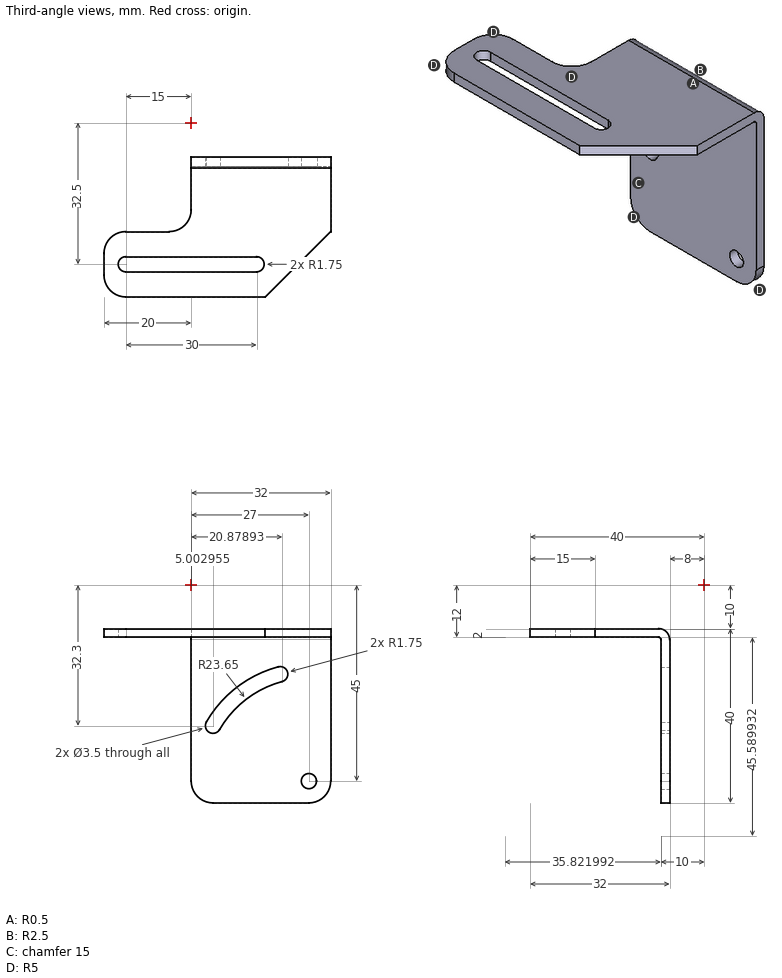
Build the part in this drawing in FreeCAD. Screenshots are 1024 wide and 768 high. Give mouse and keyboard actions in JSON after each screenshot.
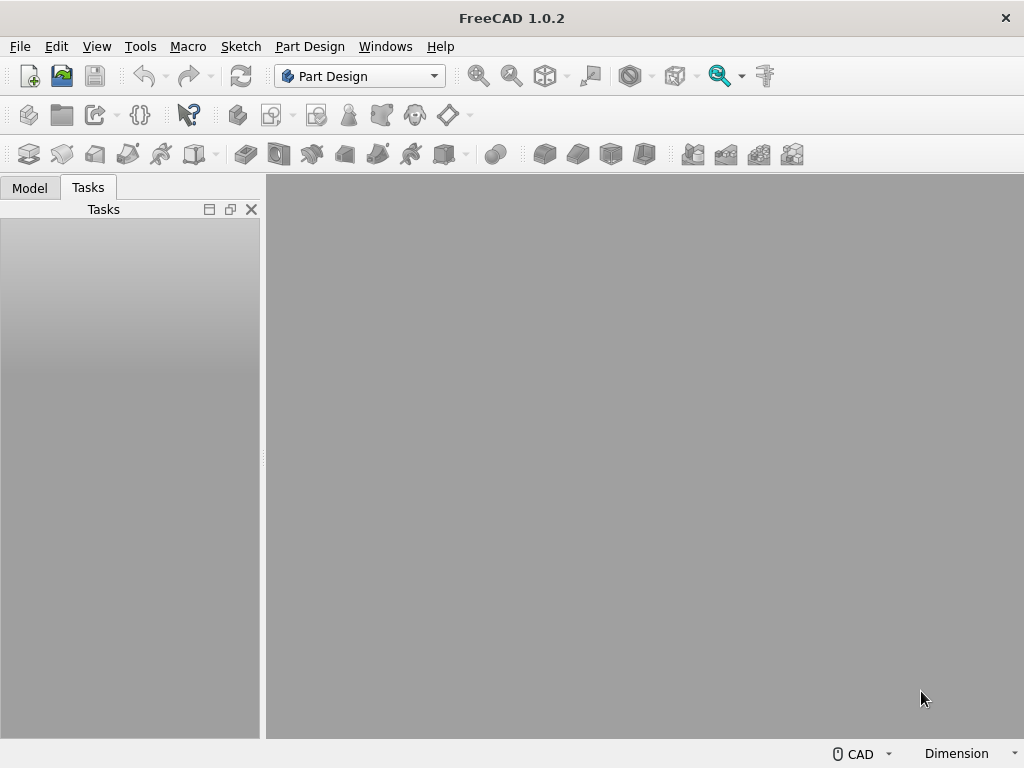
{"action": "left_click", "coordinate": [29, 76]}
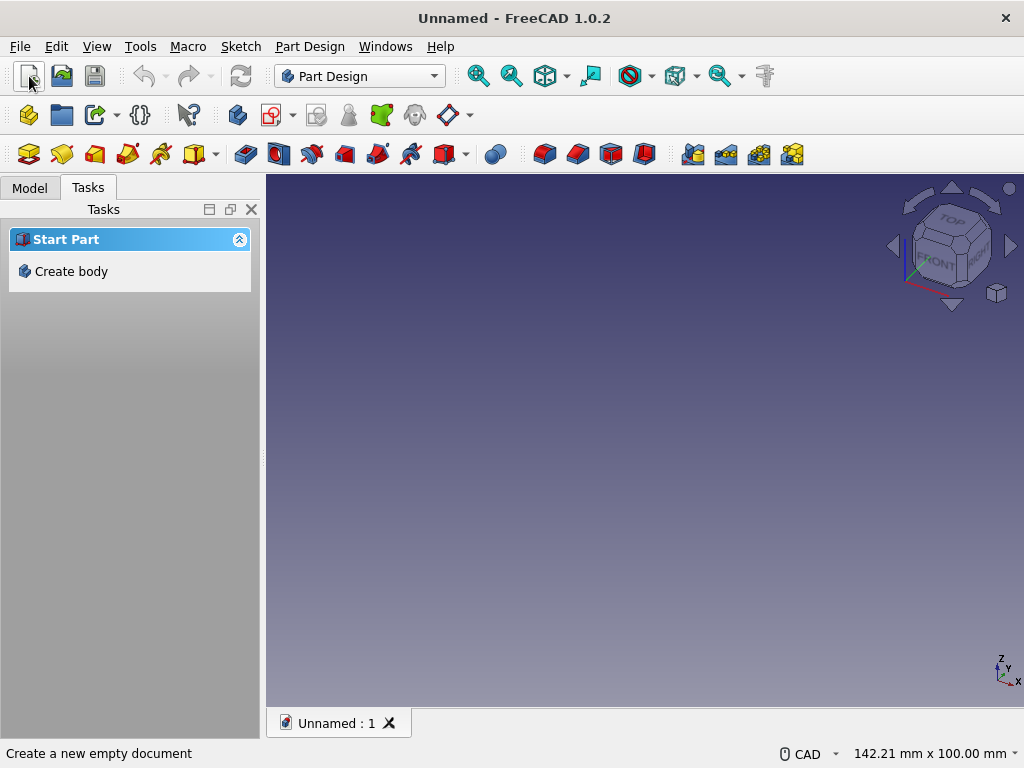
{"action": "left_click", "coordinate": [270, 116]}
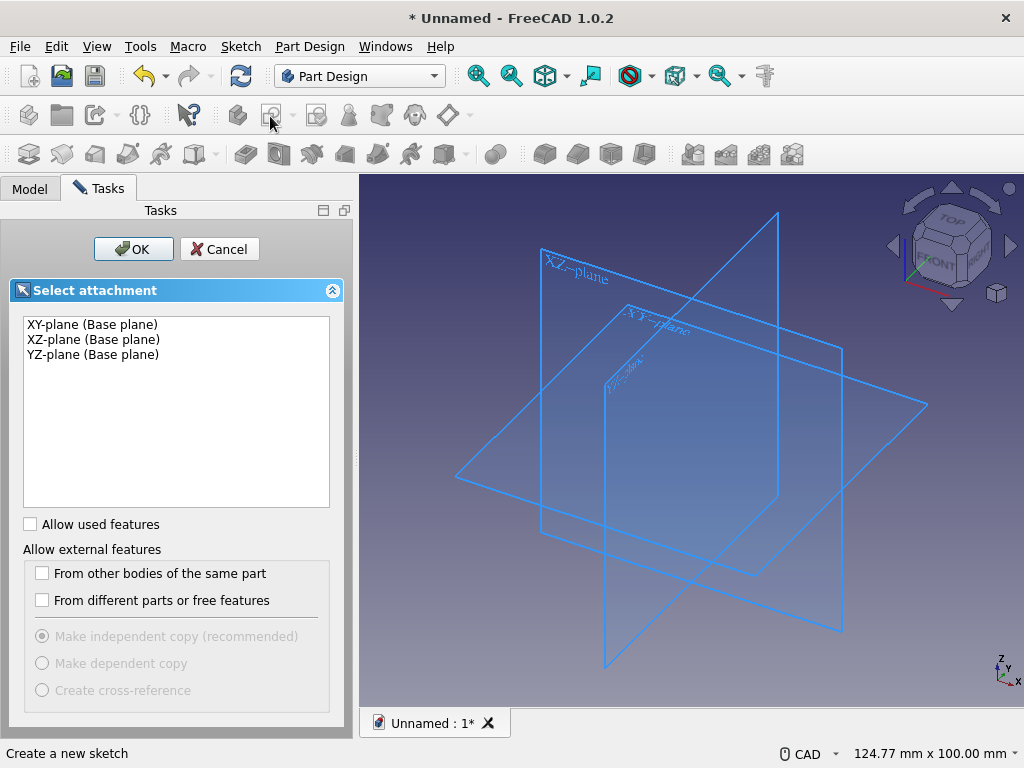
{"action": "left_click", "coordinate": [84, 354]}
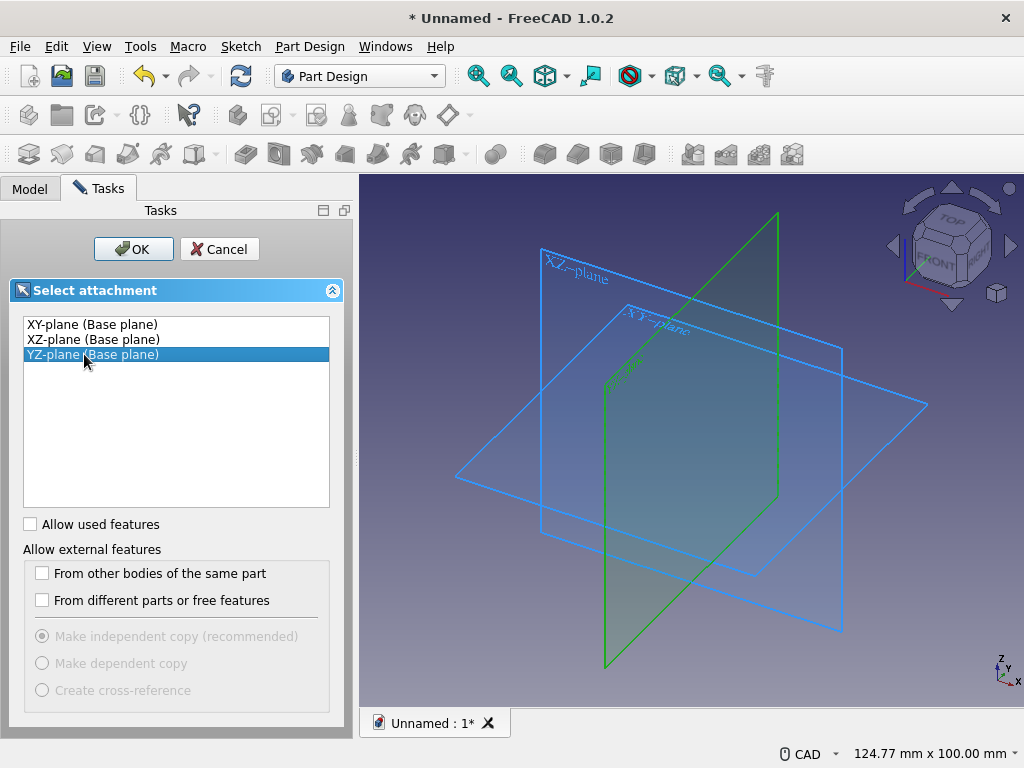
{"action": "left_click", "coordinate": [134, 249]}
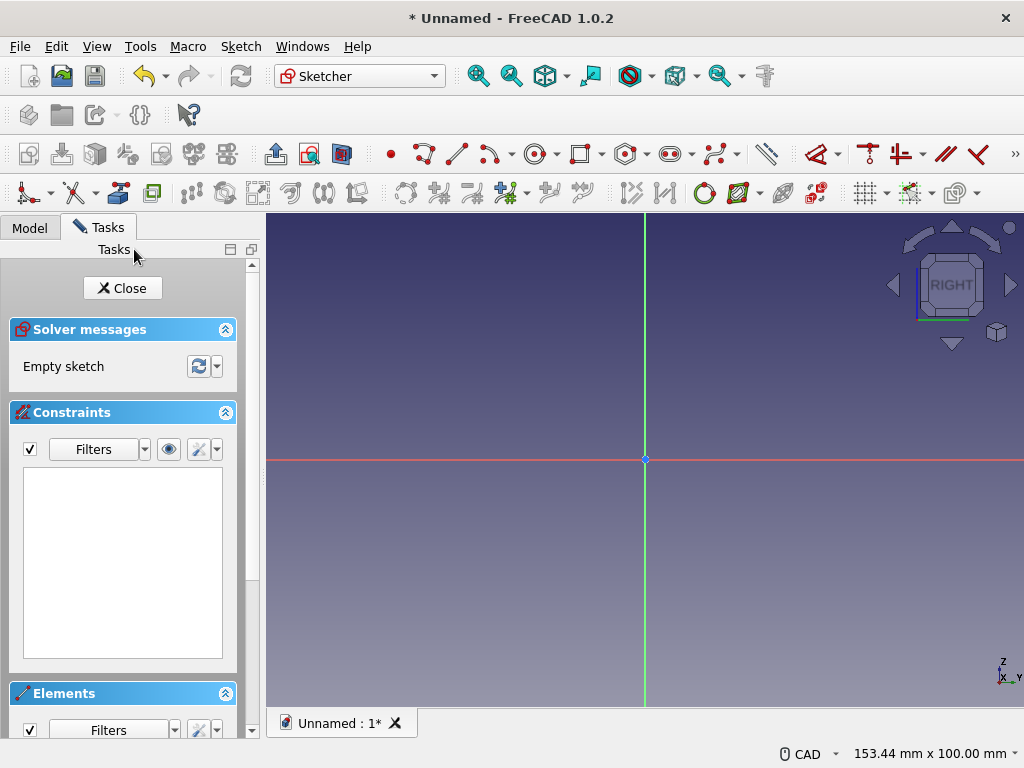
{"action": "scroll", "coordinate": [713, 241], "scroll_direction": "down", "scroll_amount": 1}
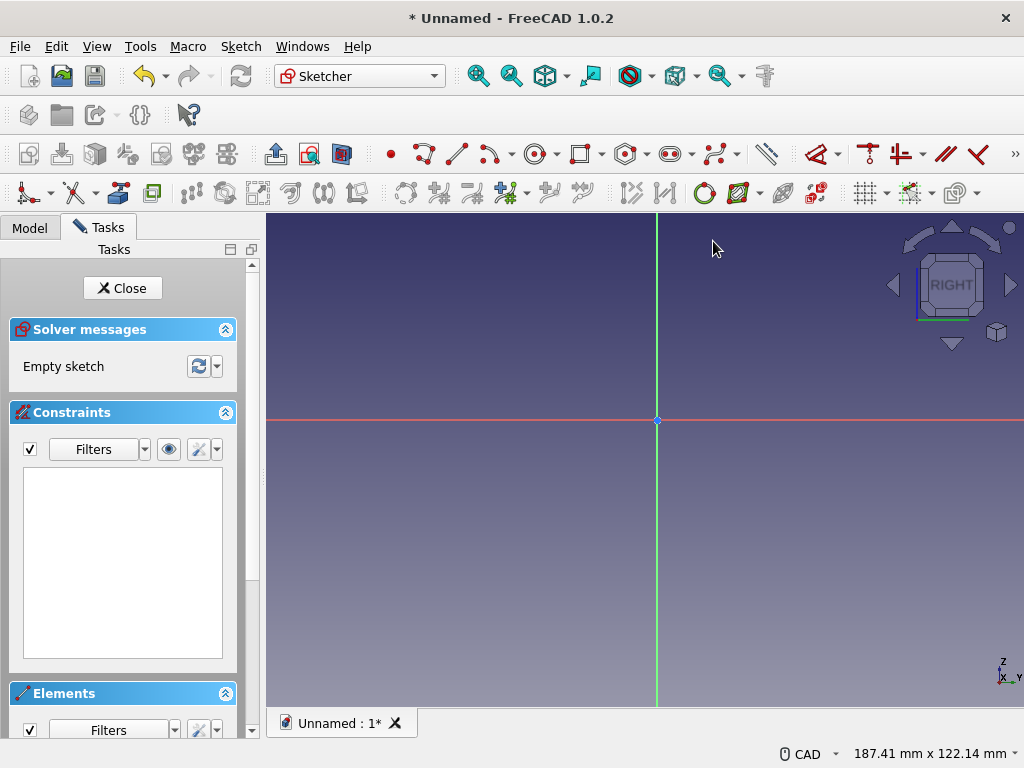
{"action": "scroll", "coordinate": [577, 646], "scroll_direction": "up", "scroll_amount": 2}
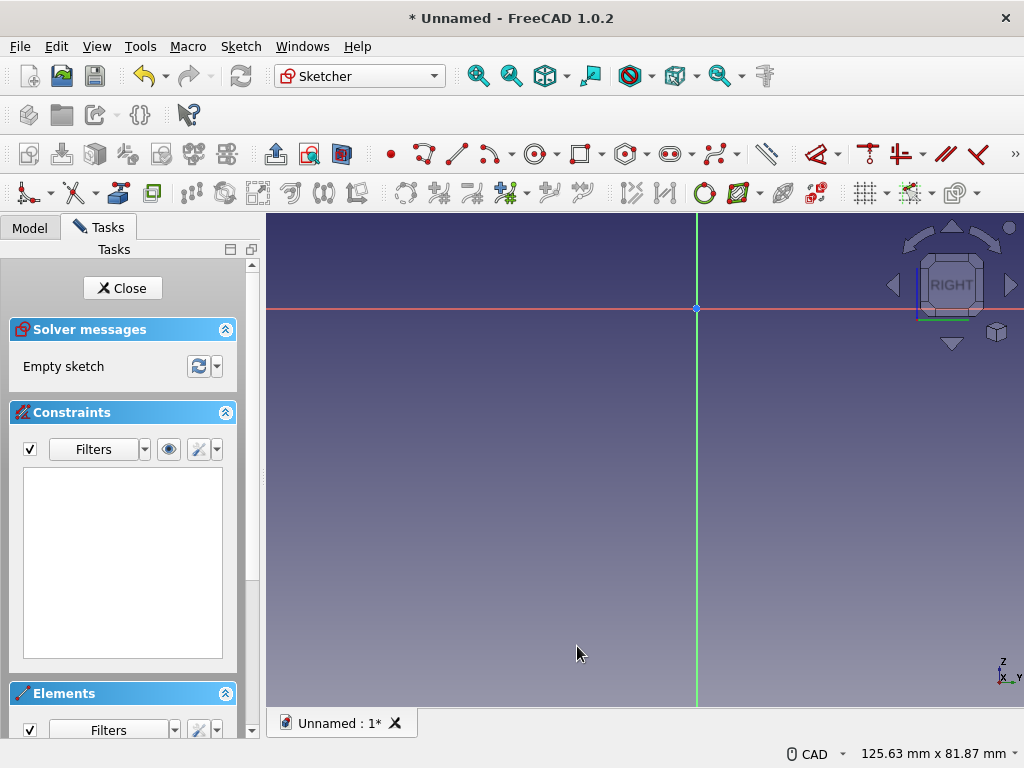
{"action": "key", "text": "g r"}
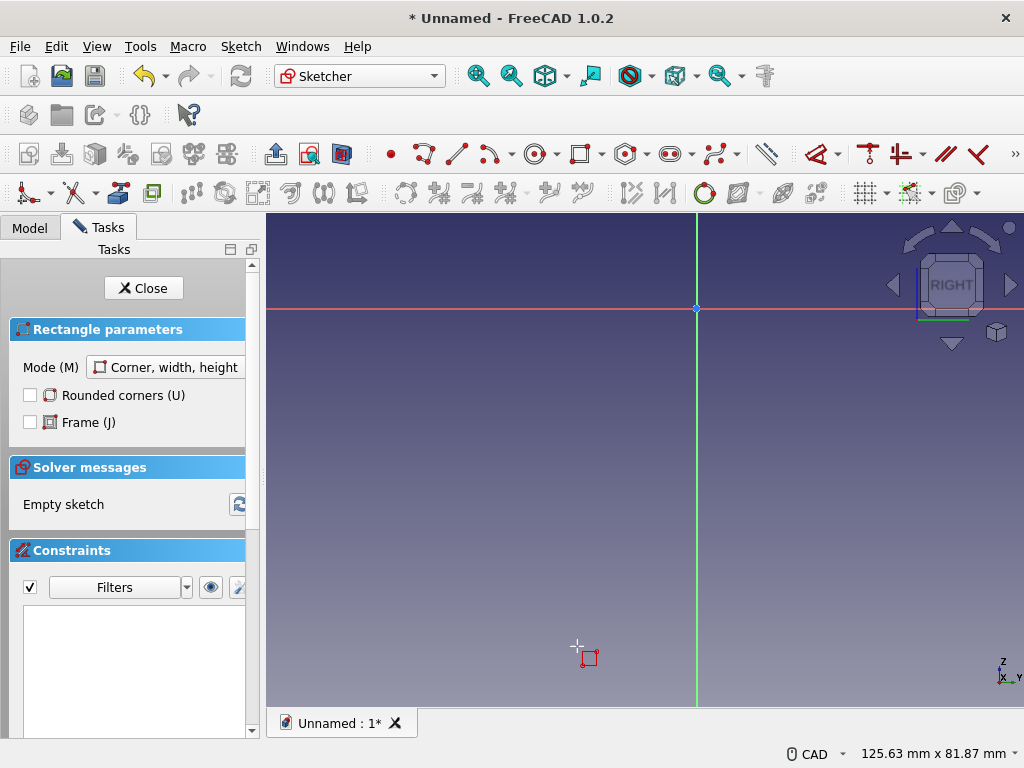
{"action": "left_click", "coordinate": [455, 369]}
{"action": "mouse_move", "coordinate": [649, 611]}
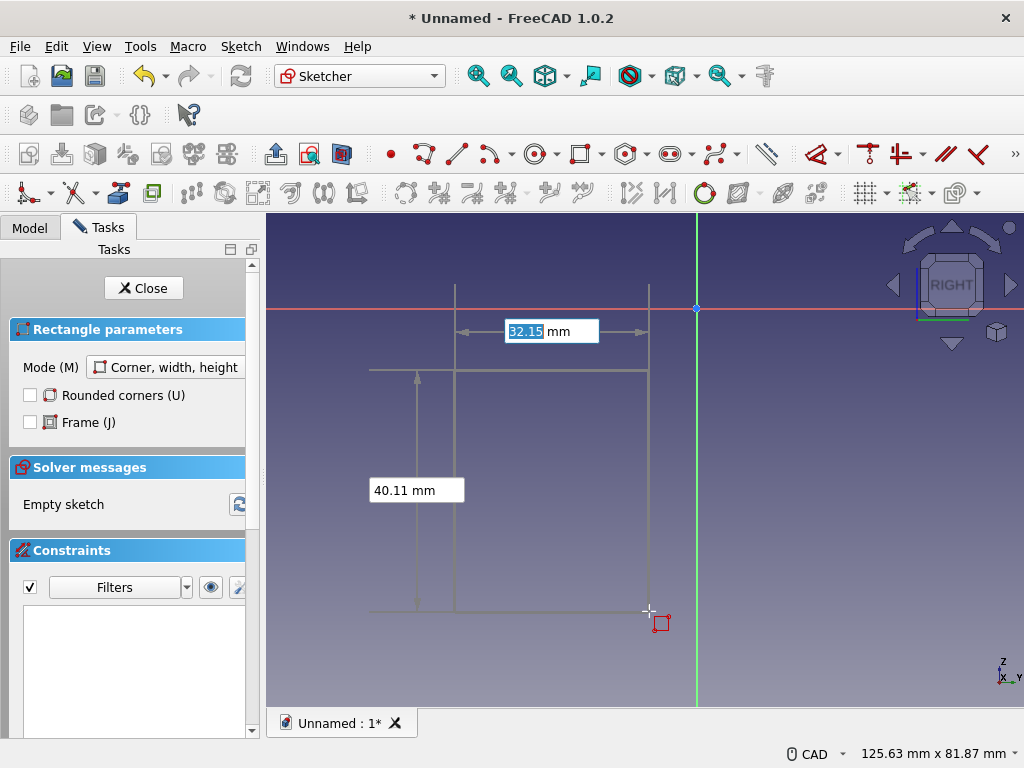
{"action": "type", "text": "32"}
{"action": "key", "text": "Tab"}
{"action": "type", "text": "40"}
{"action": "key", "text": "Return"}
{"action": "key", "text": "Escape"}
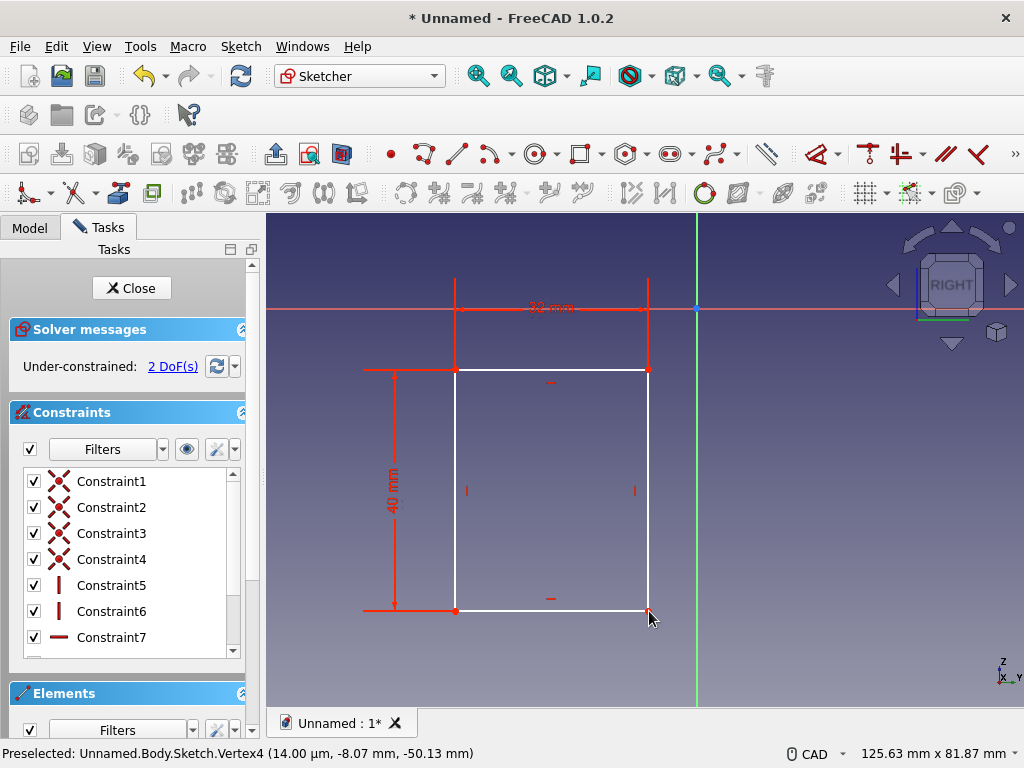
{"action": "key", "text": "d"}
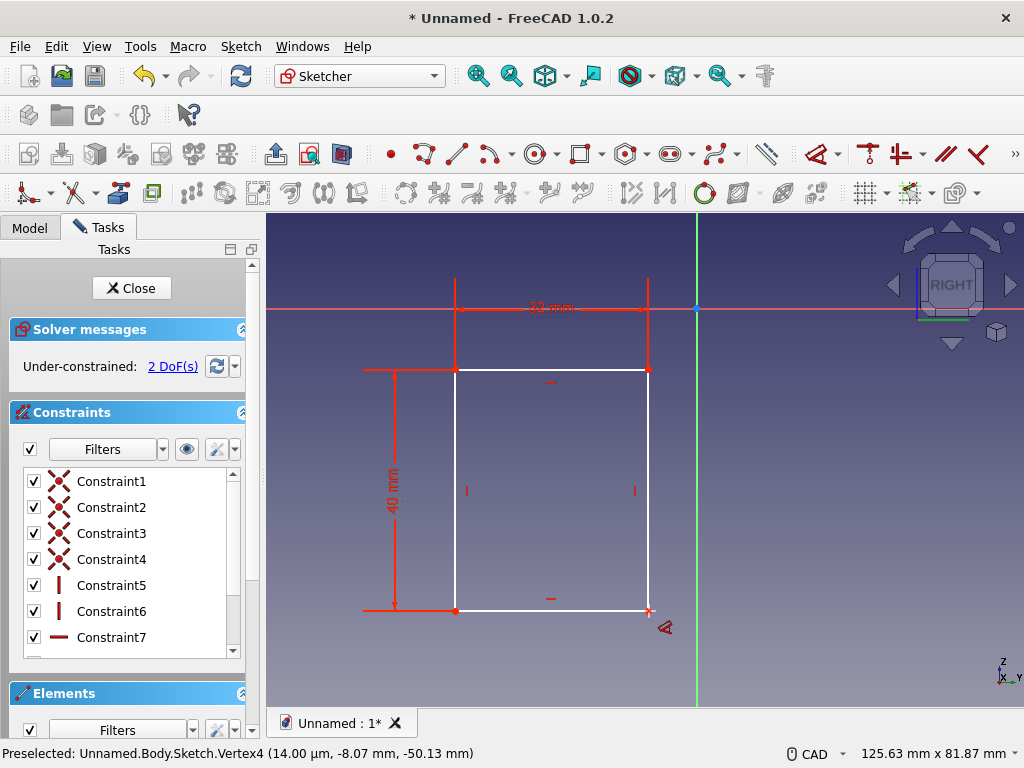
{"action": "left_click", "coordinate": [648, 611]}
{"action": "left_click", "coordinate": [672, 645]}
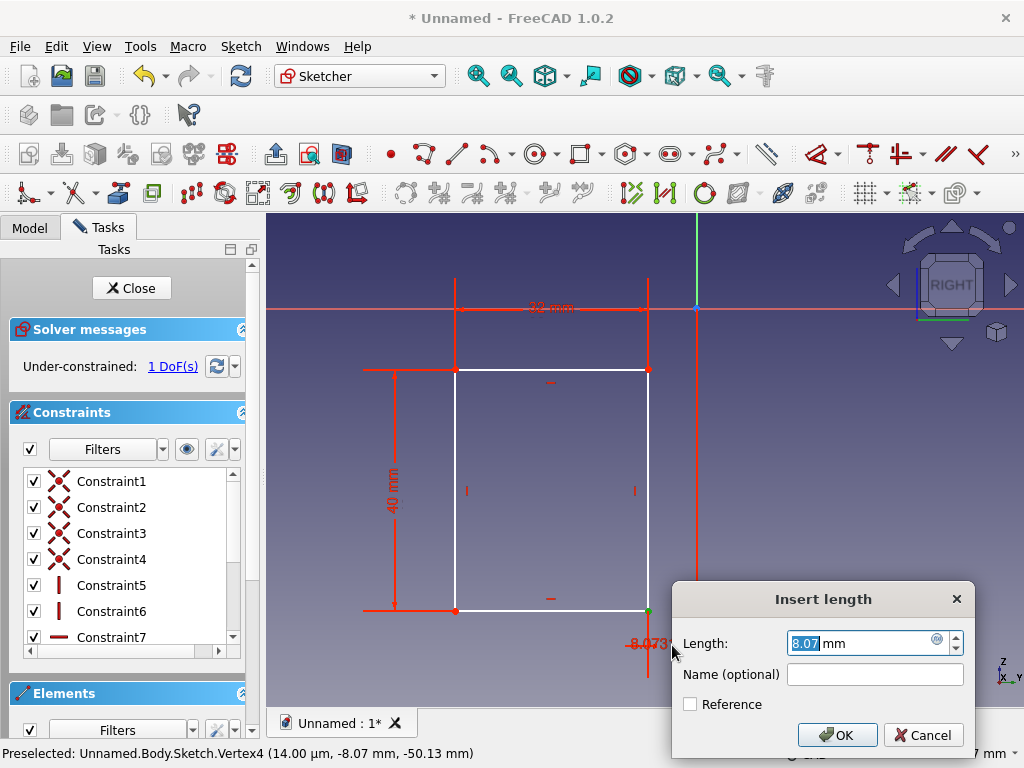
{"action": "type", "text": "8"}
{"action": "key", "text": "Return"}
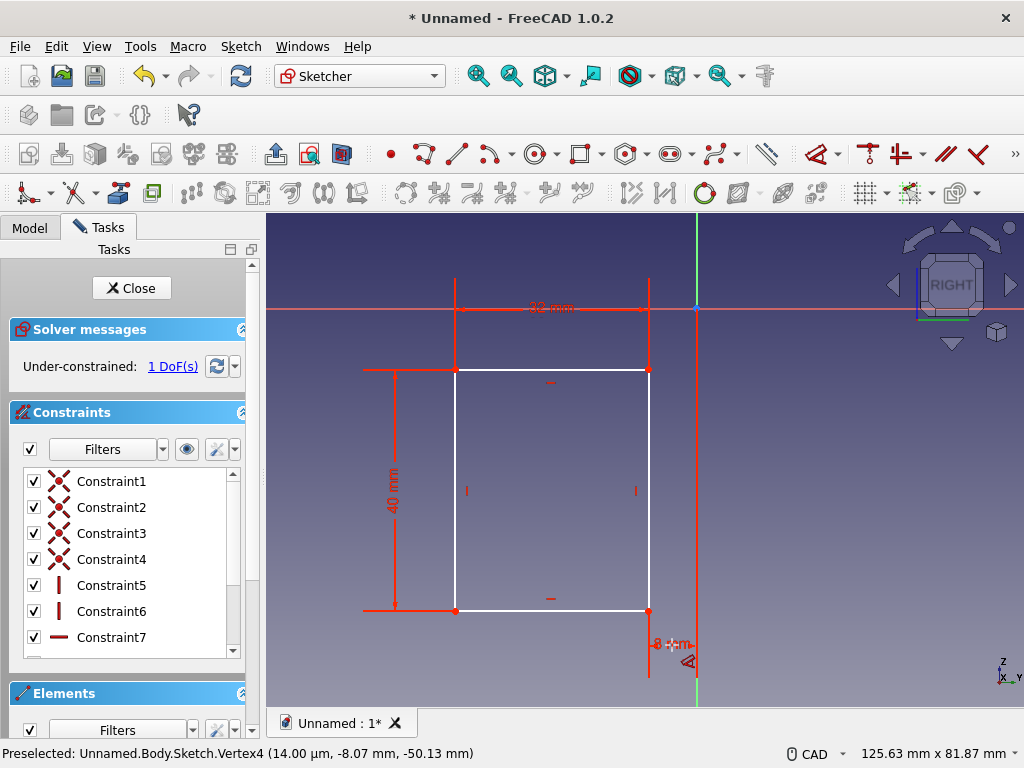
{"action": "left_click", "coordinate": [455, 370]}
{"action": "left_click", "coordinate": [421, 339]}